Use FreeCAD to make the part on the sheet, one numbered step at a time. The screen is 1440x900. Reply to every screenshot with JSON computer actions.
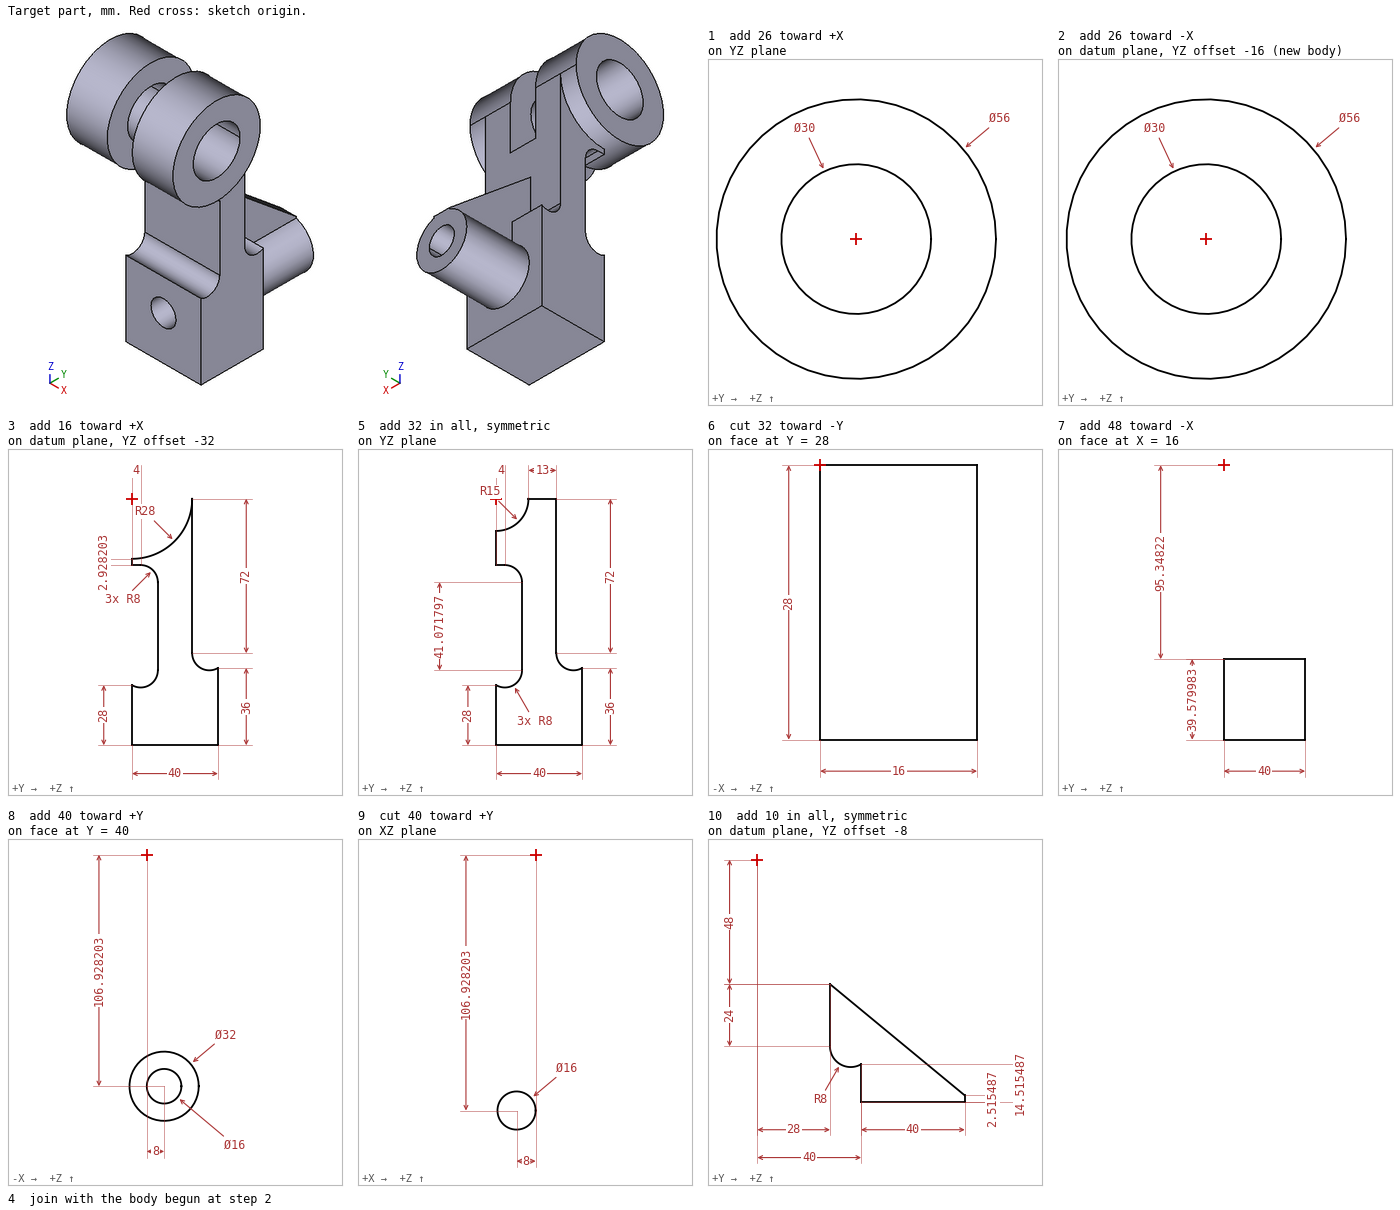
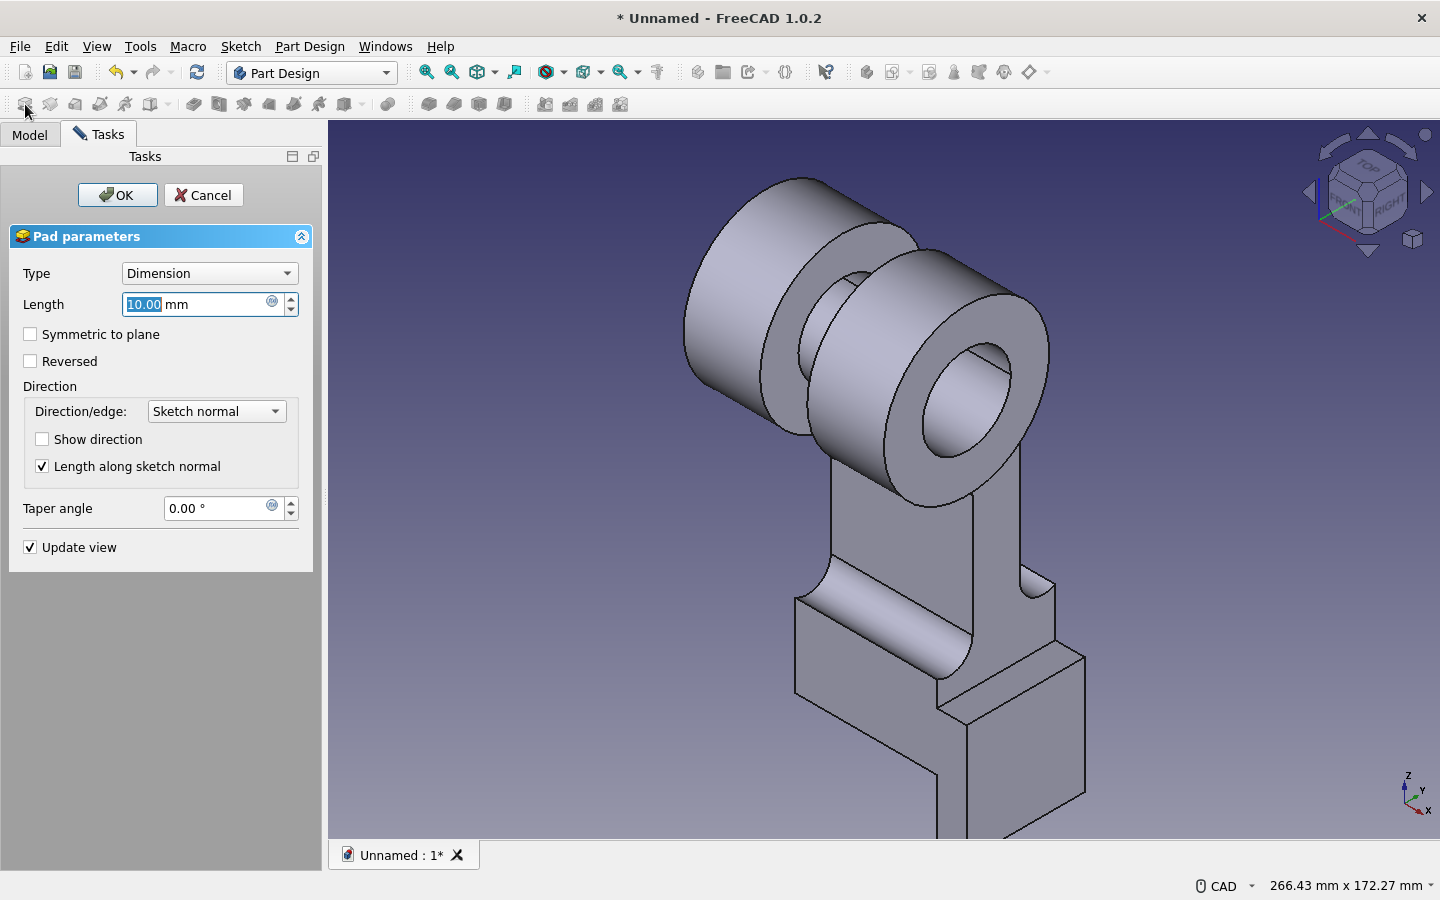
{"action": "type", "text": "48"}
{"action": "key", "text": "Tab"}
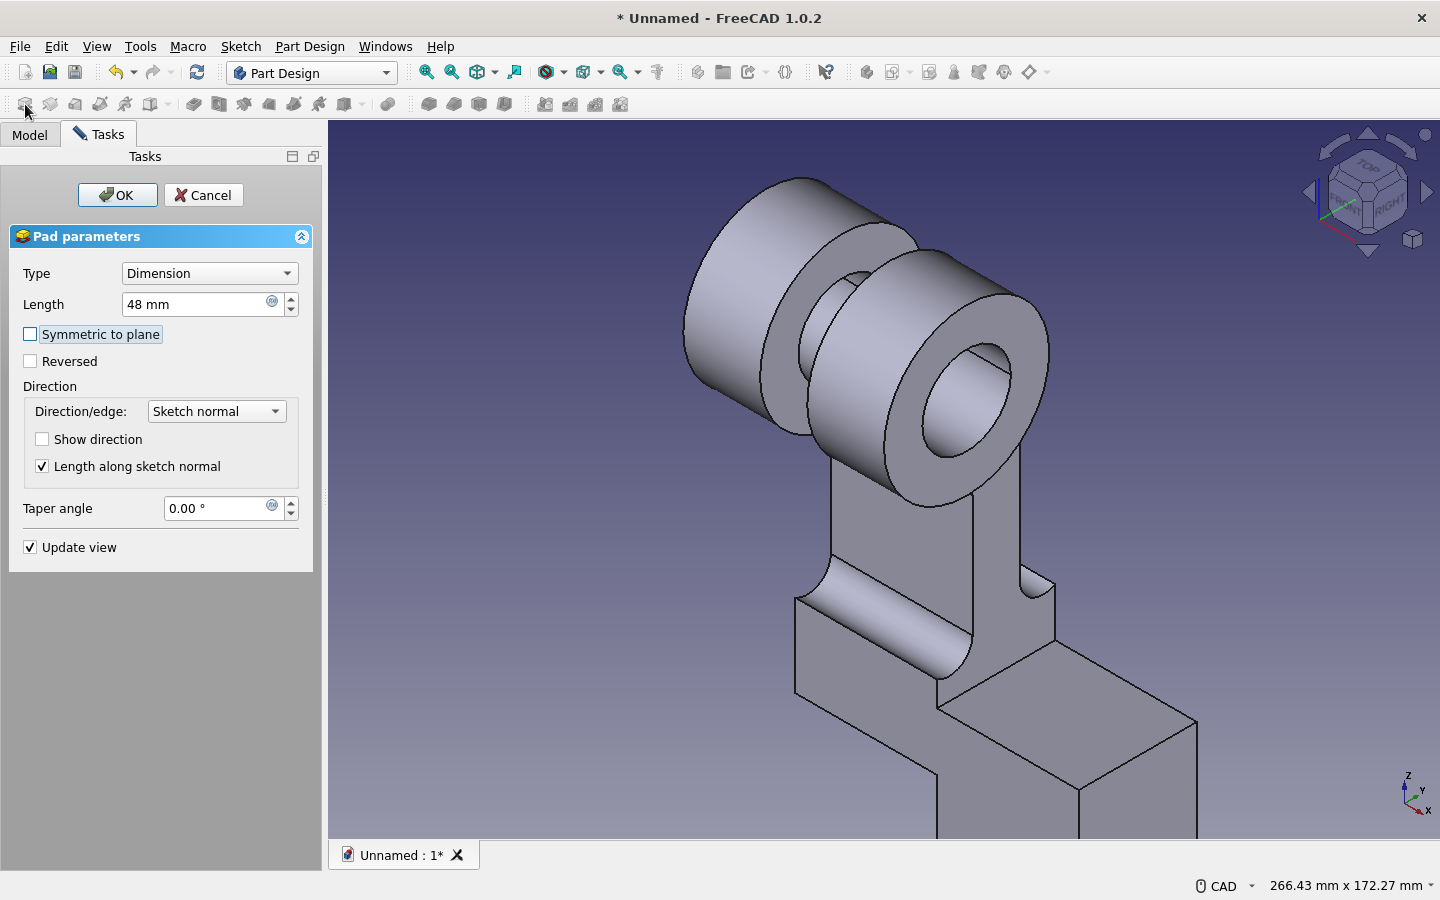
{"action": "left_click", "coordinate": [31, 361]}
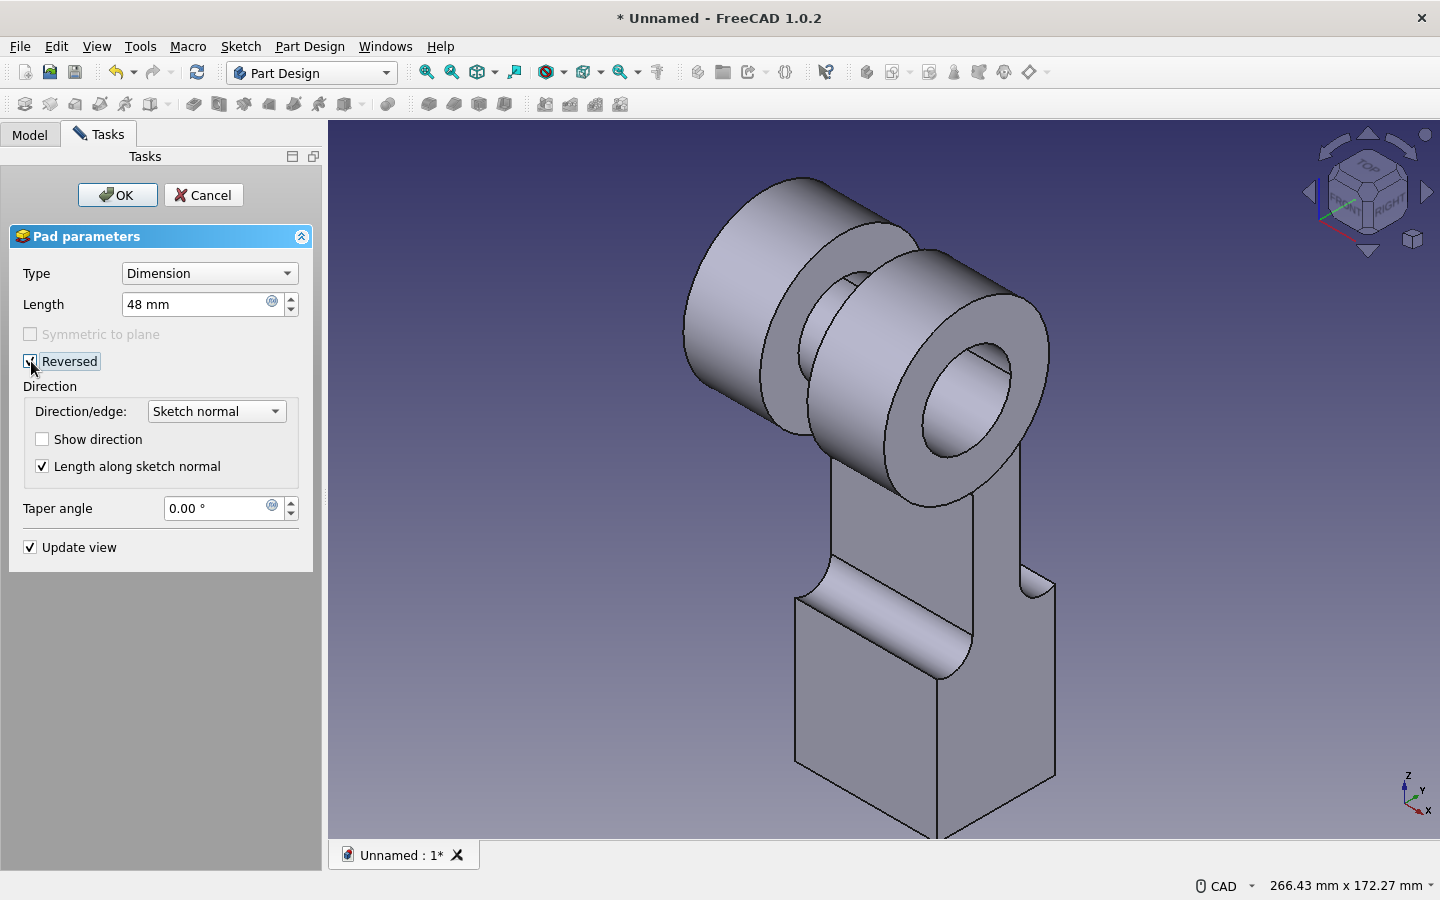
{"action": "left_click", "coordinate": [118, 195]}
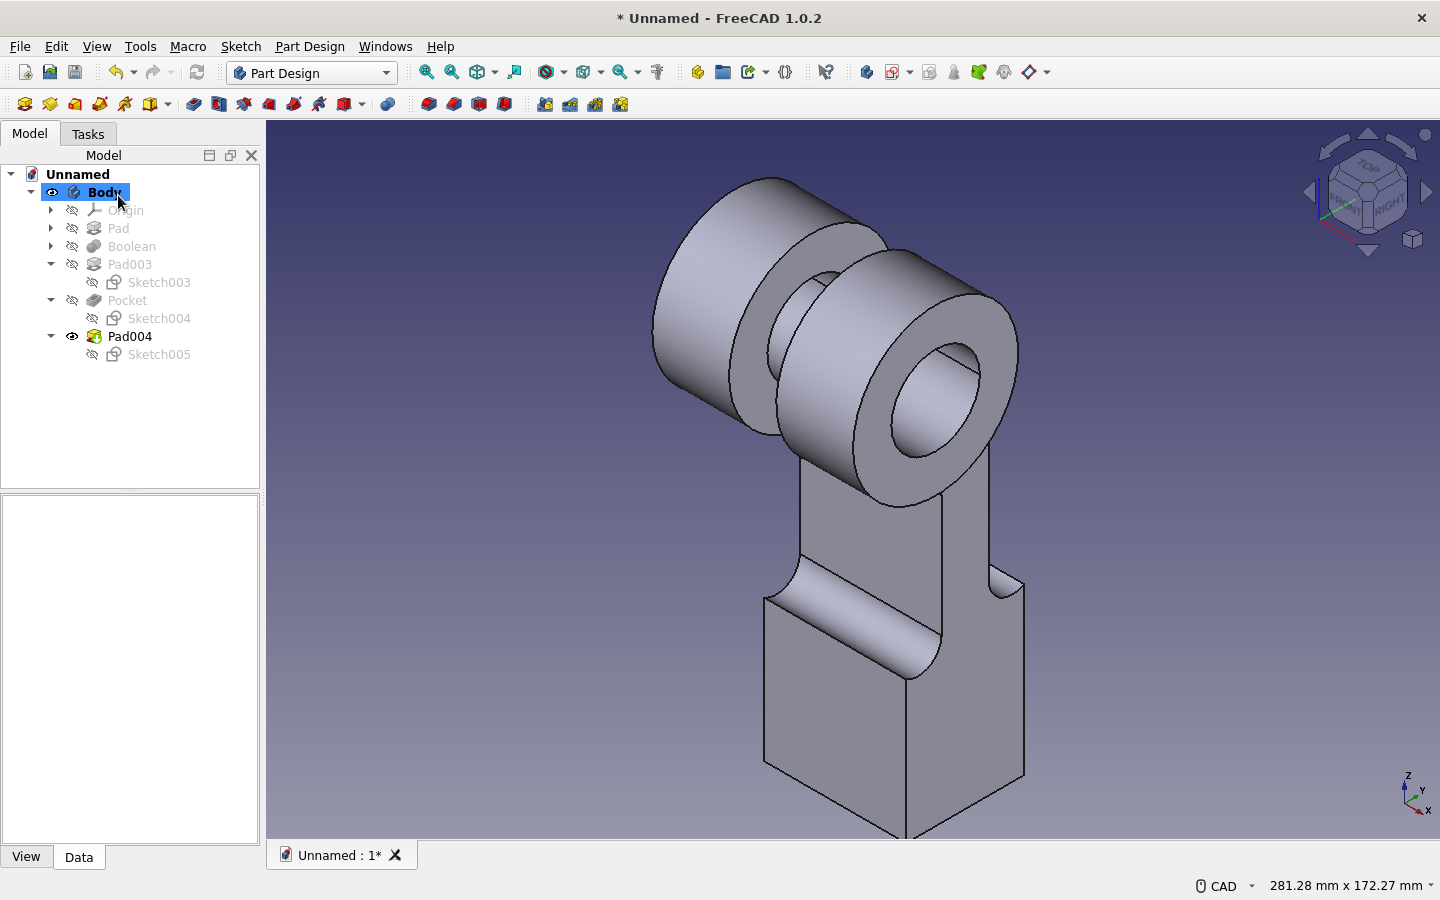
{"action": "left_click", "coordinate": [427, 72]}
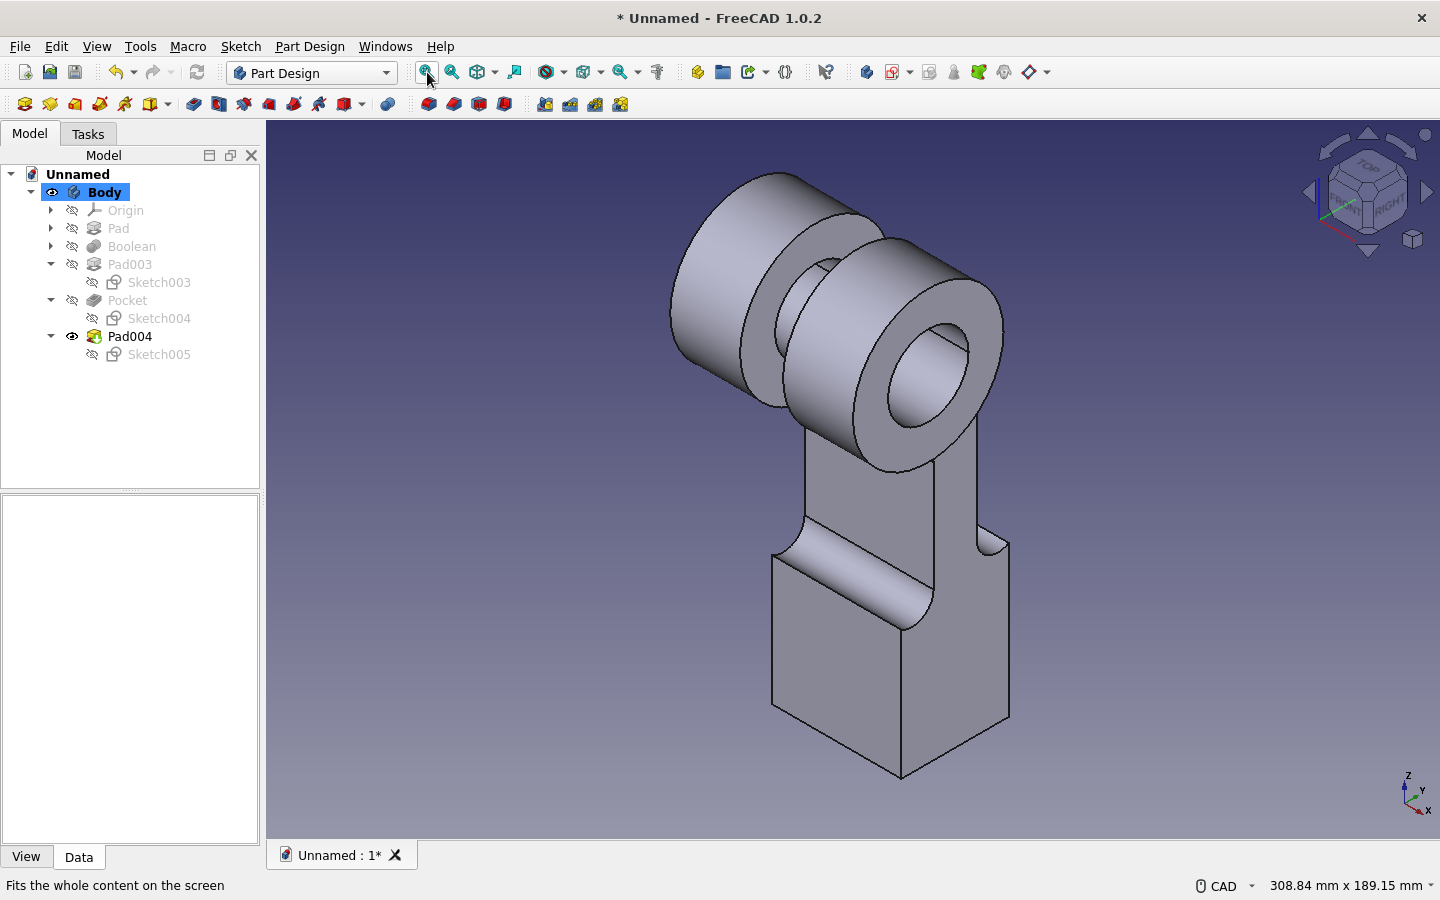
{"action": "key", "text": "4"}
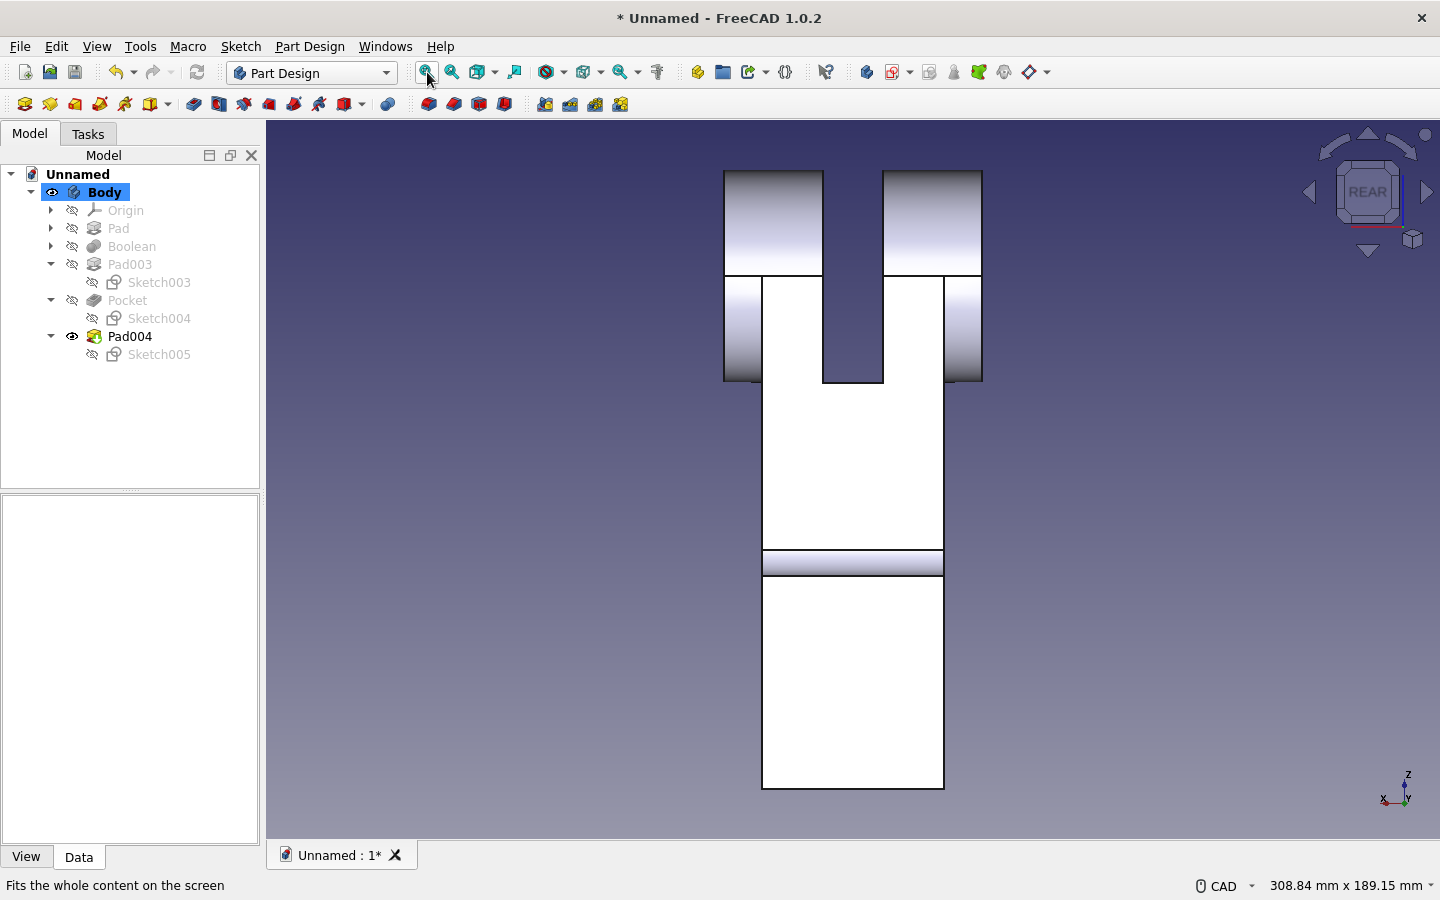
{"action": "left_click", "coordinate": [853, 682]}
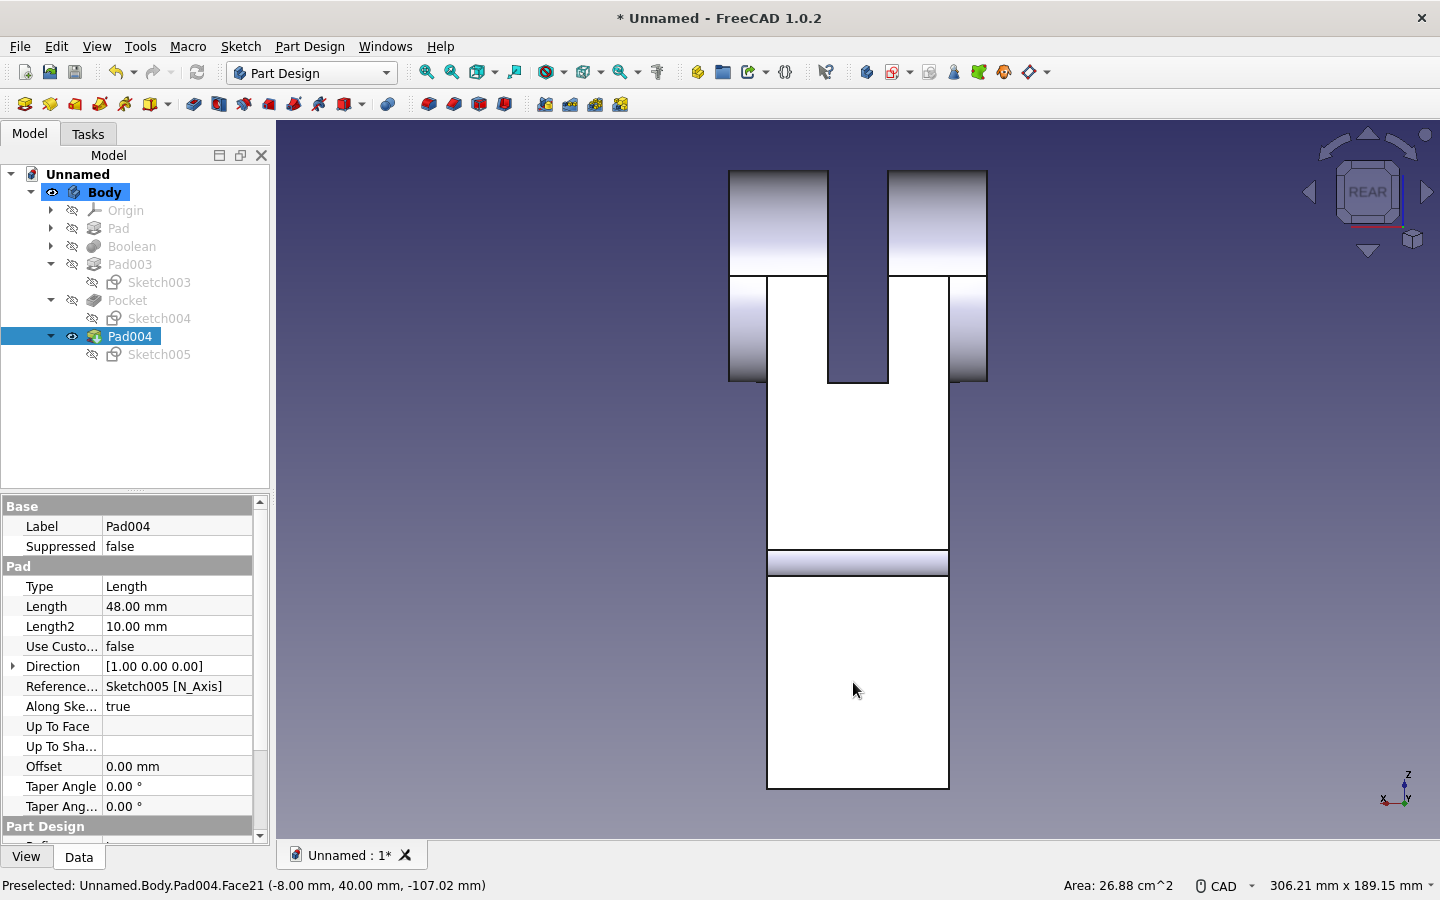
{"action": "left_click", "coordinate": [892, 72]}